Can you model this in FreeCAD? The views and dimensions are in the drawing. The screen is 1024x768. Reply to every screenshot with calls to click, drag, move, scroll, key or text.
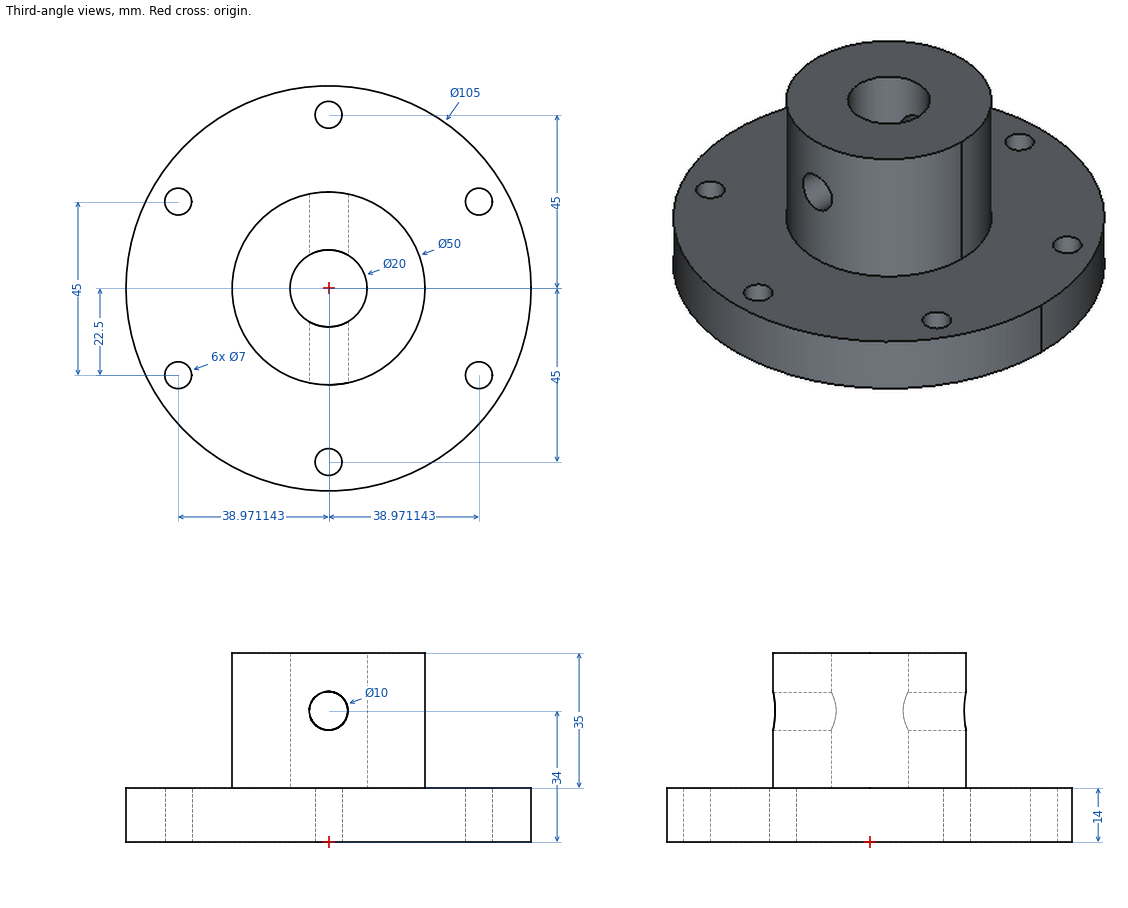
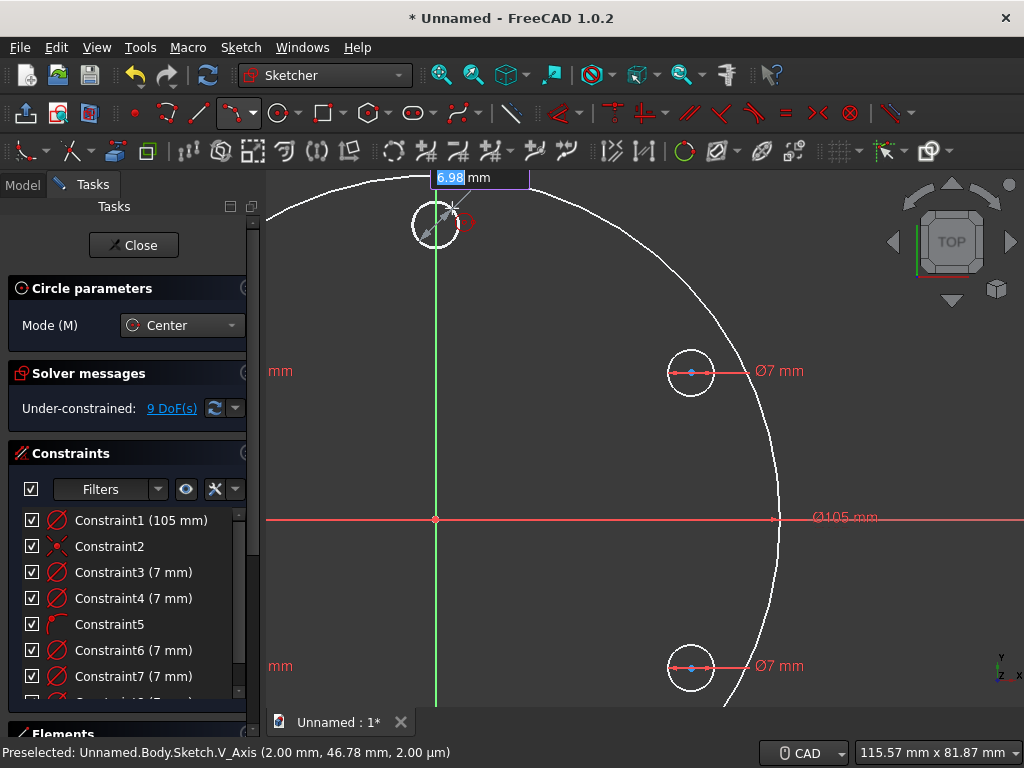
text(7)
key(Return)
key(Escape)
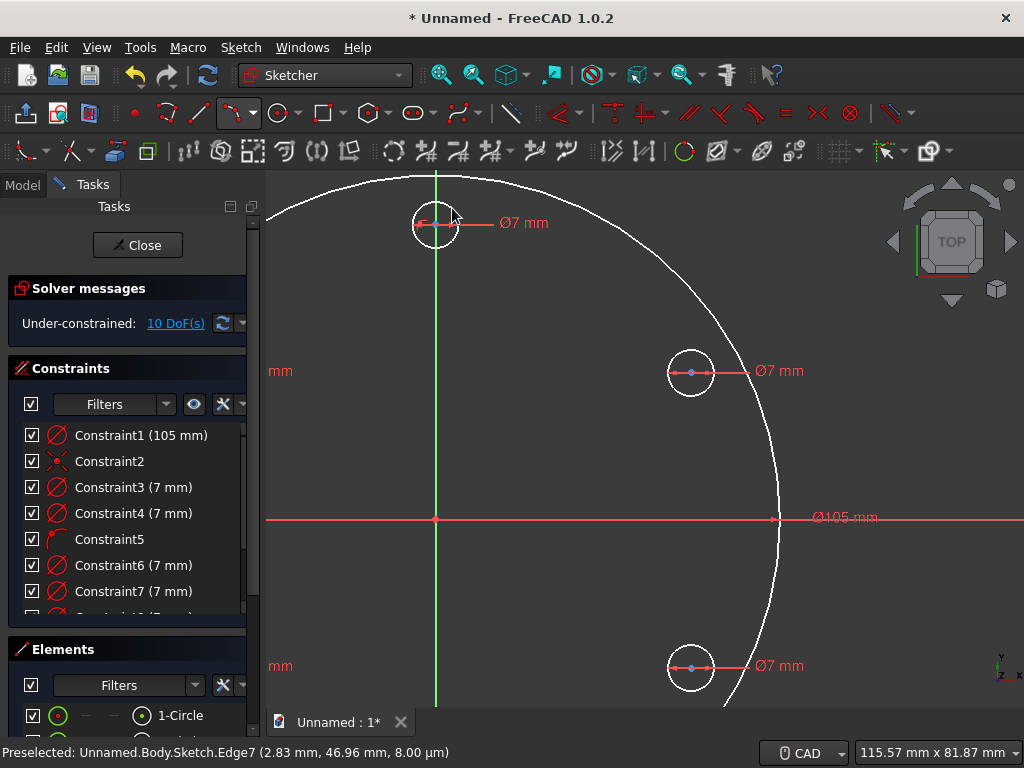
scroll(691, 372, down, 4)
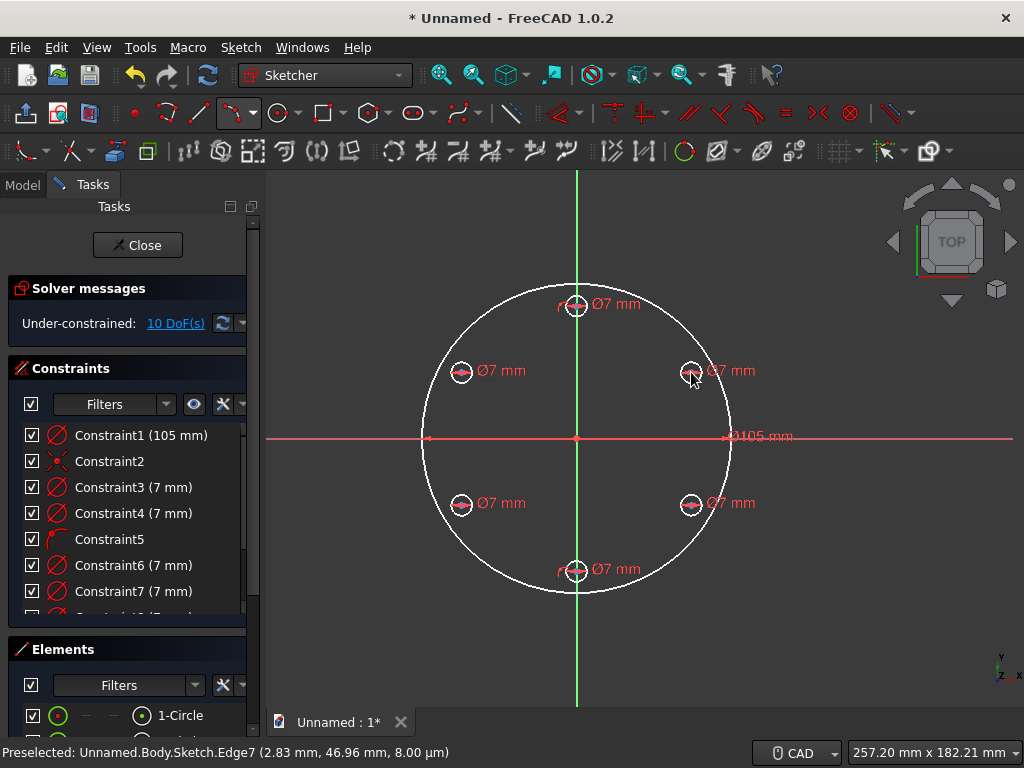
click(462, 505)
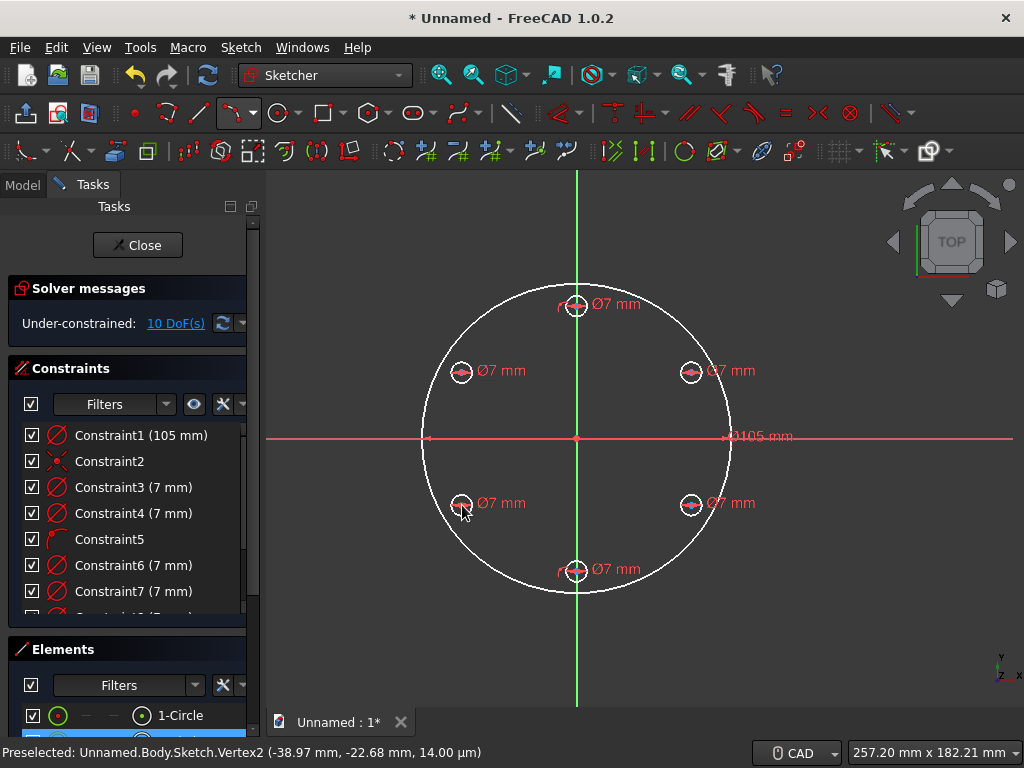
click(691, 505)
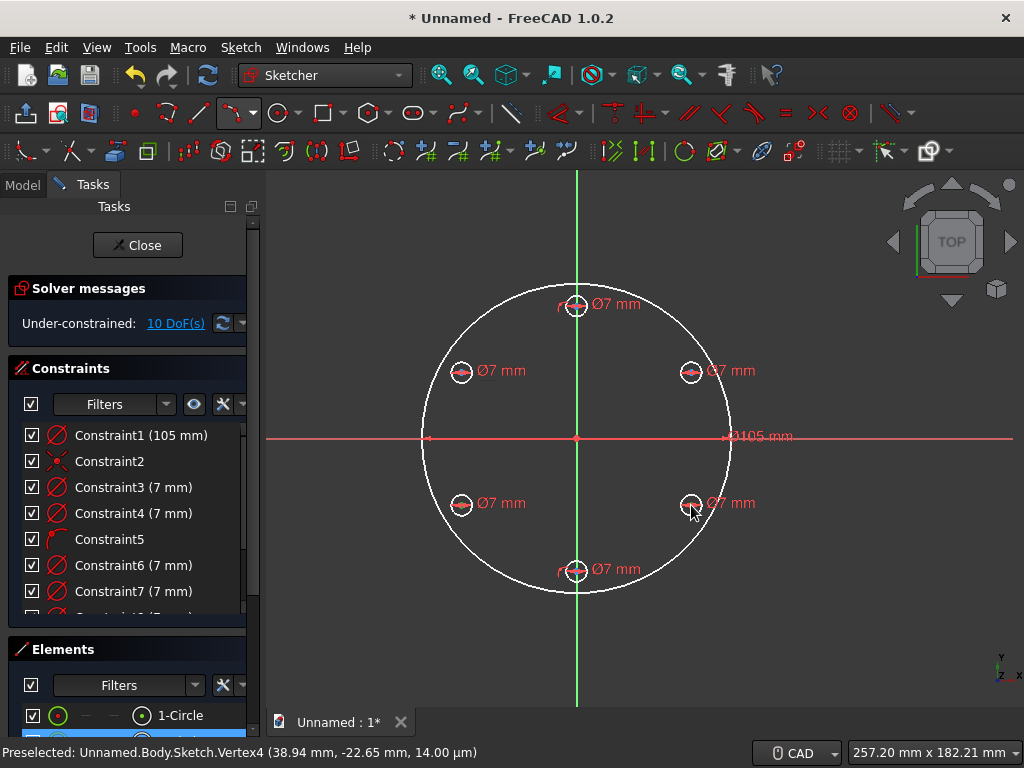
key(h)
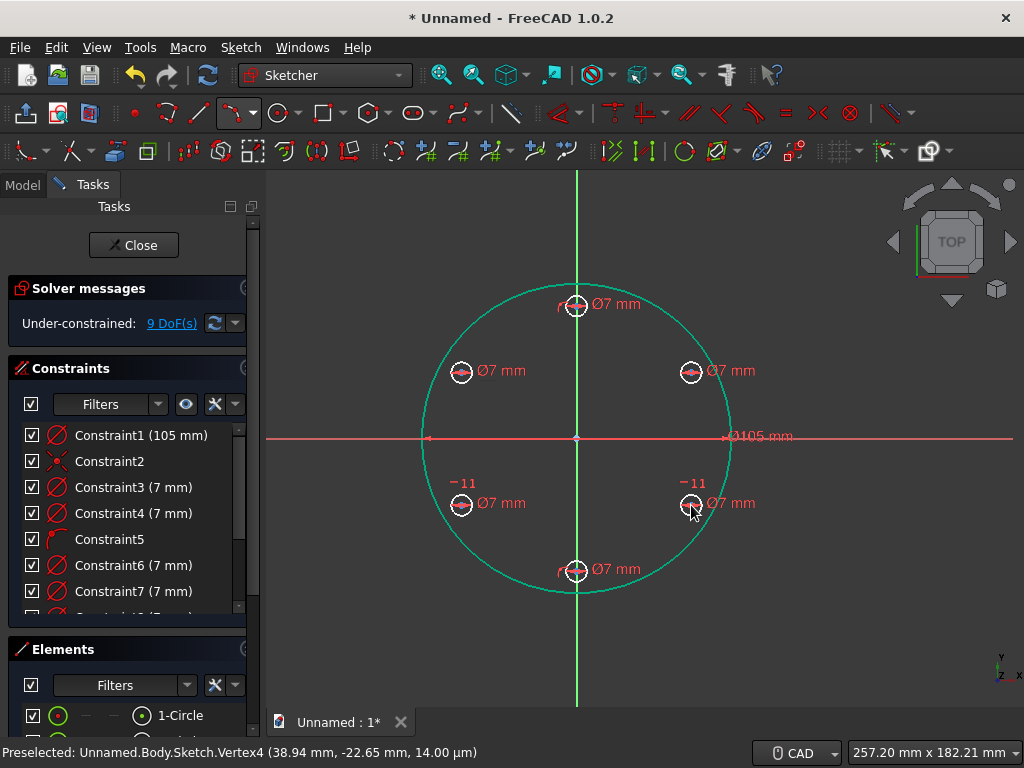
click(462, 505)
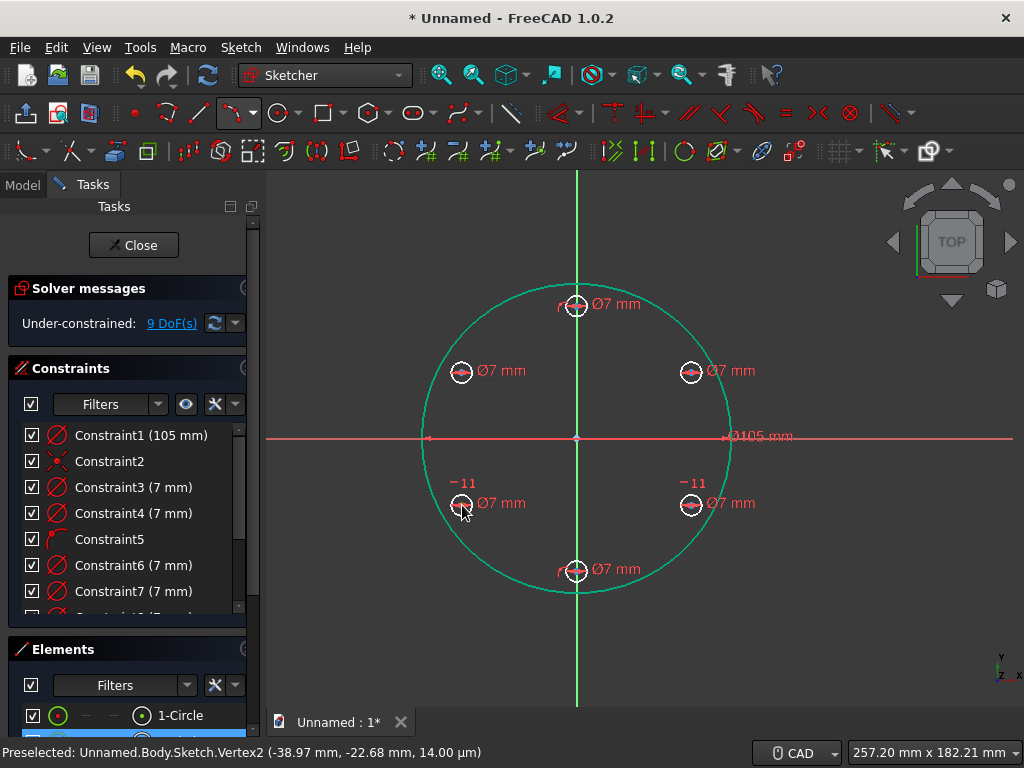
click(462, 373)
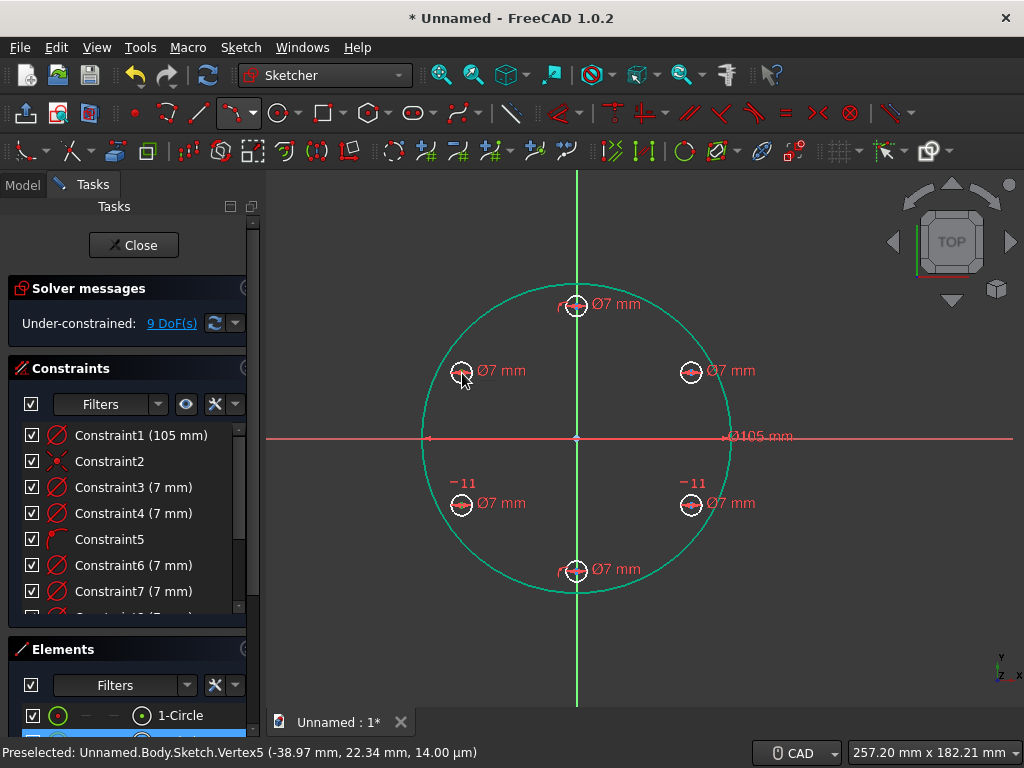
click(668, 114)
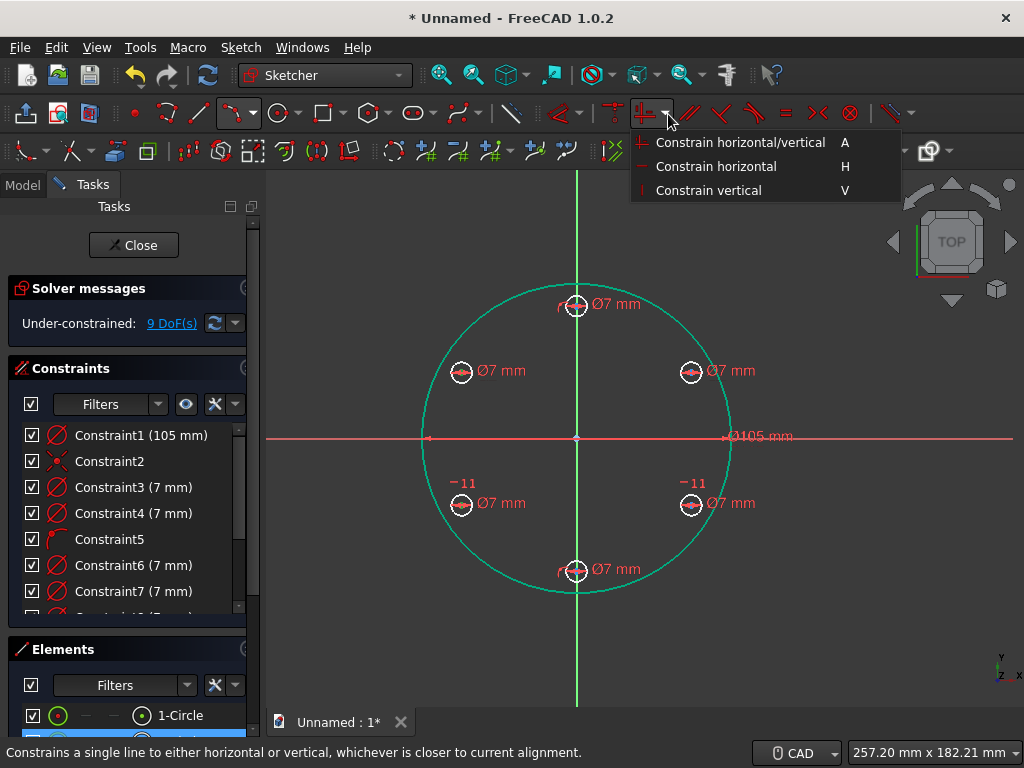
click(766, 190)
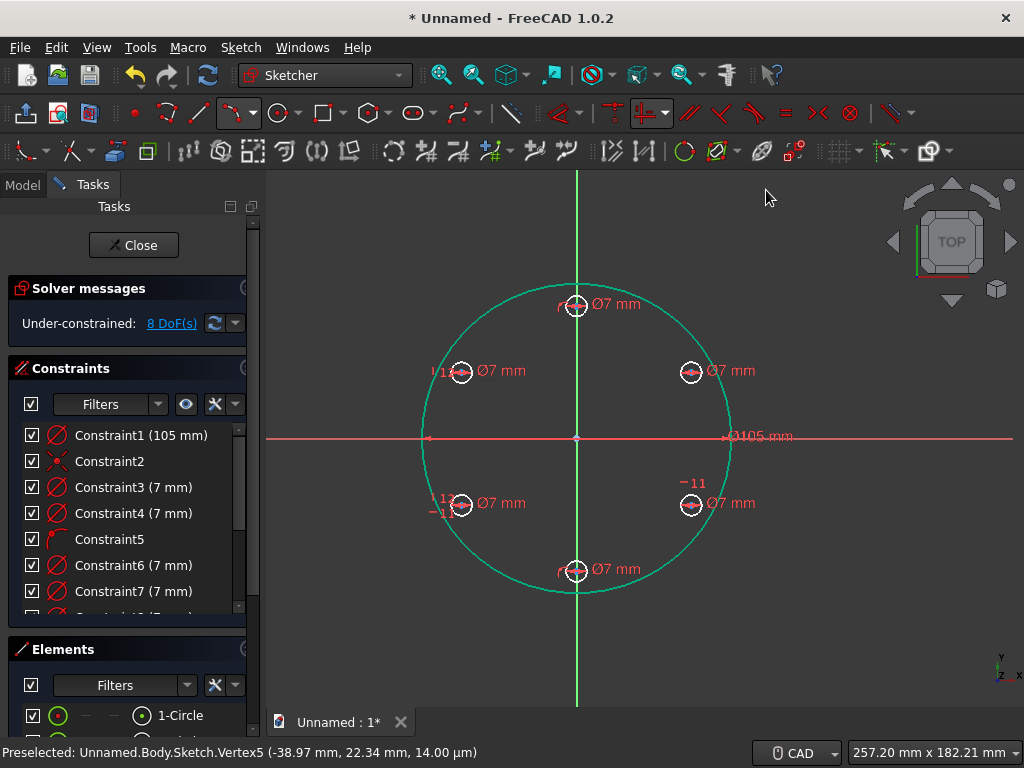
click(691, 505)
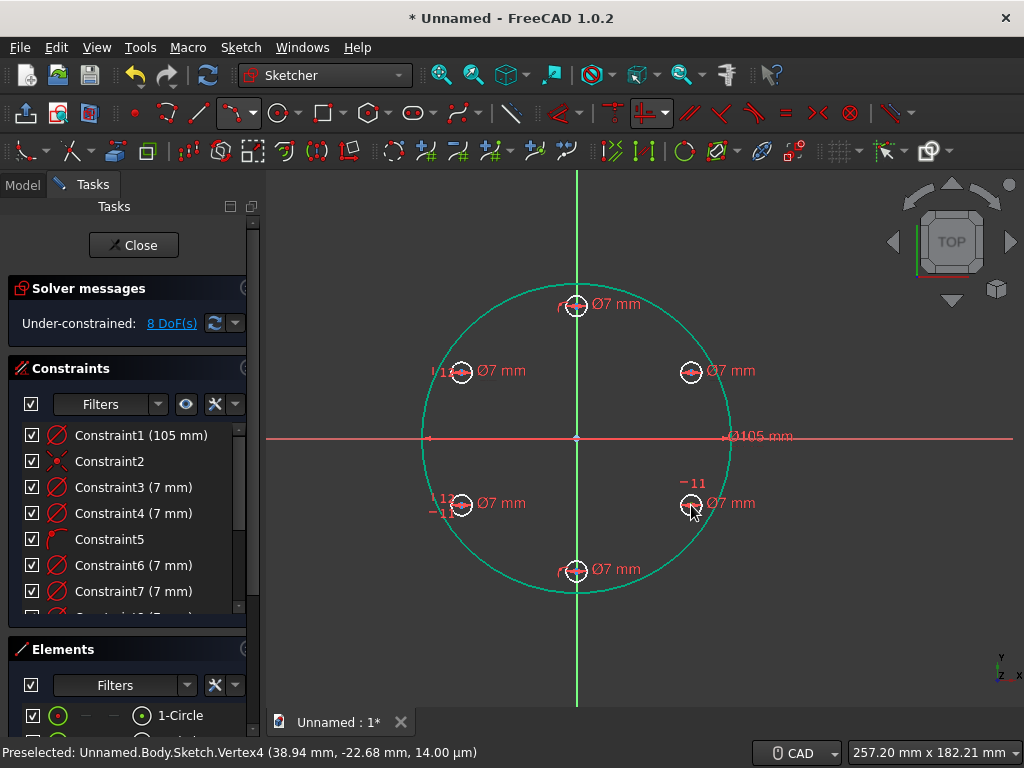
click(691, 373)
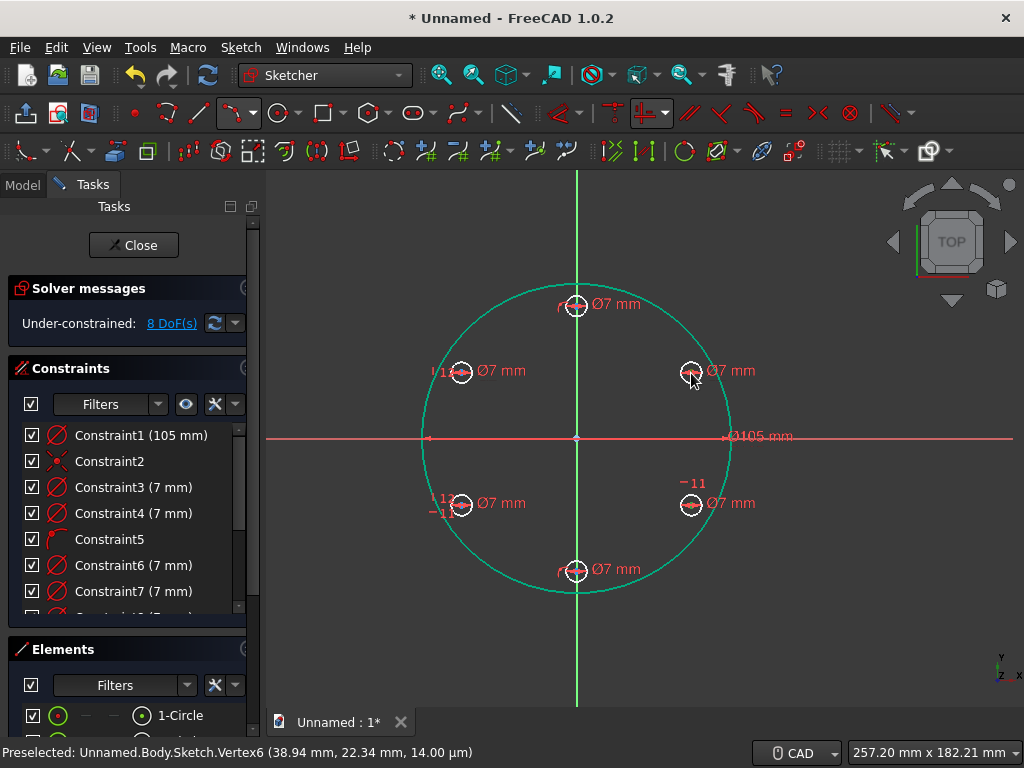
key(v)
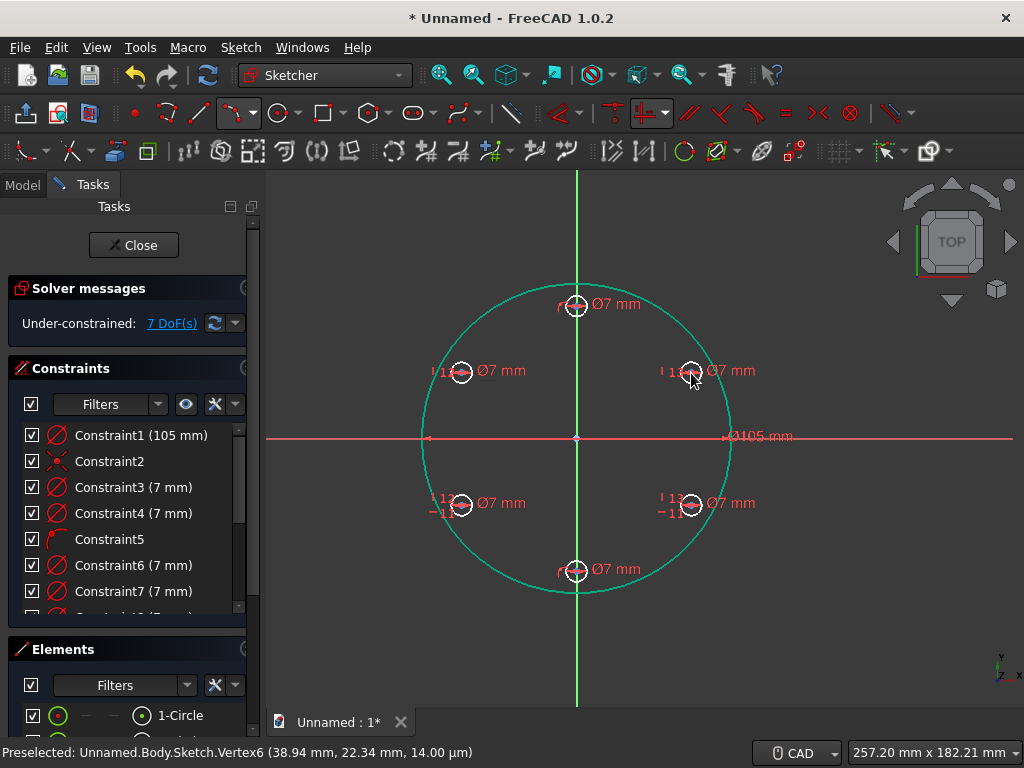
click(462, 373)